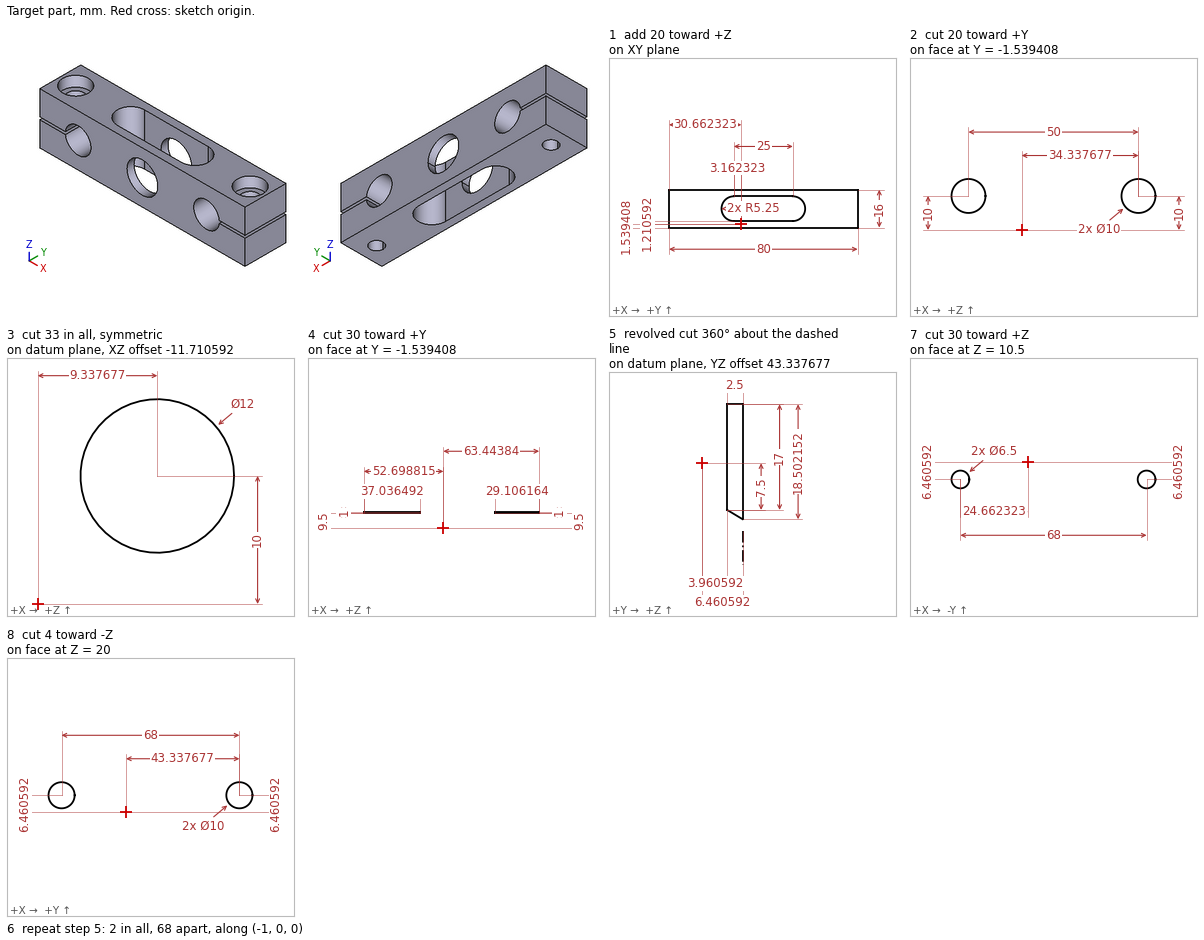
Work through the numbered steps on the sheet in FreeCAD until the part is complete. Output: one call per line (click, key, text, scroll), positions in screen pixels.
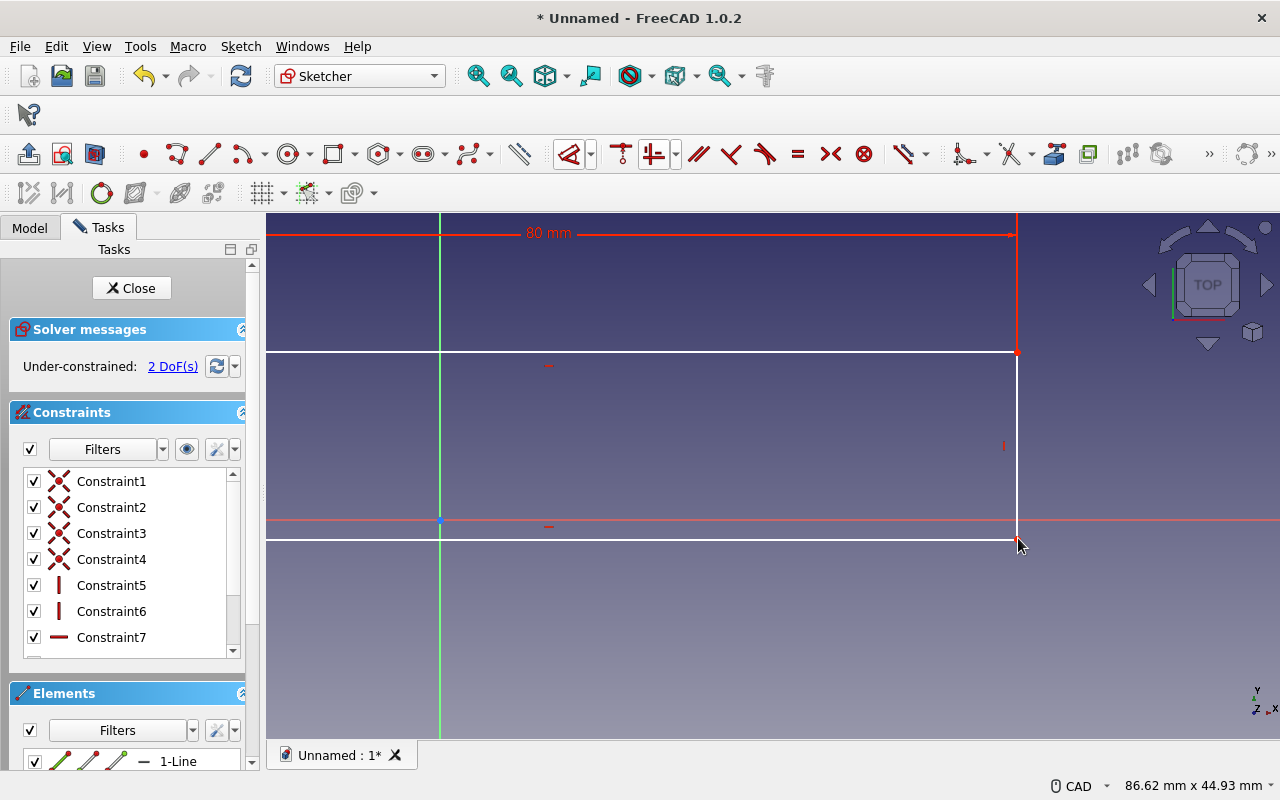
click(403, 444)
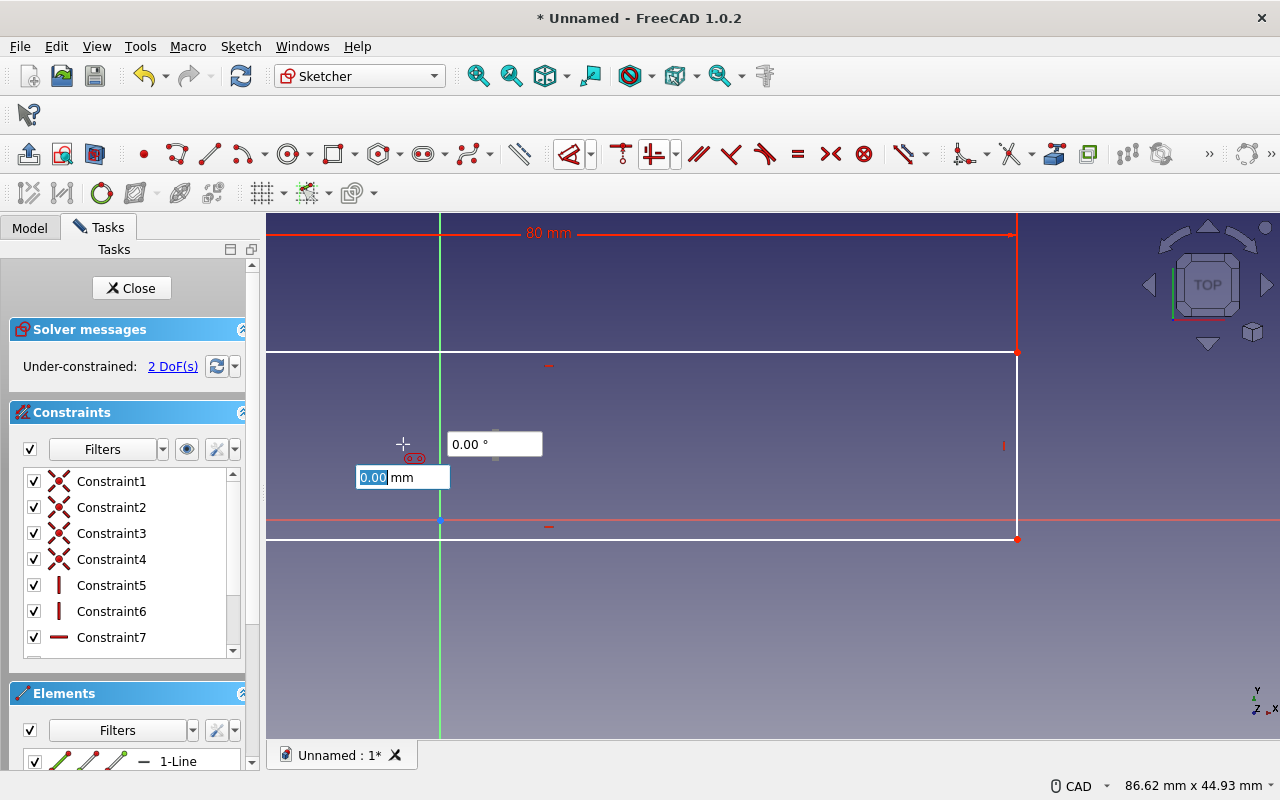
click(696, 444)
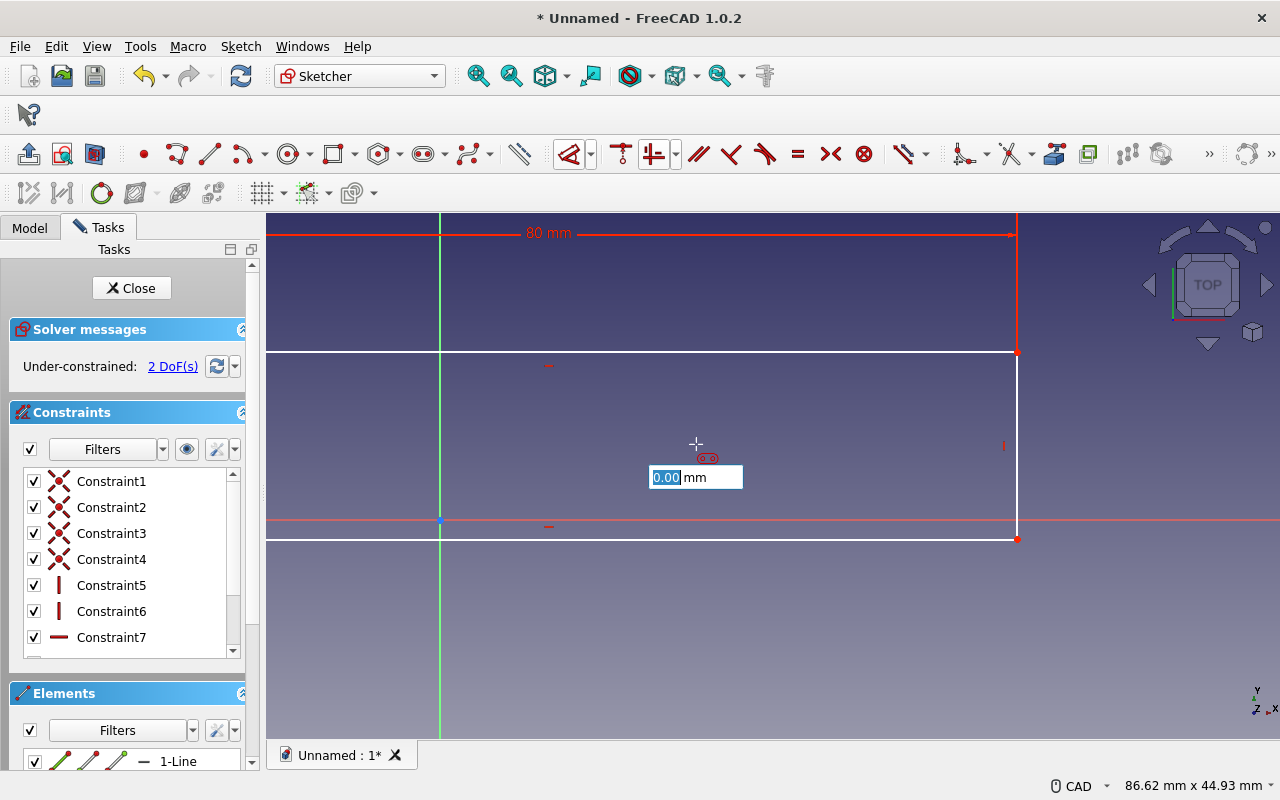
click(550, 383)
key(Escape)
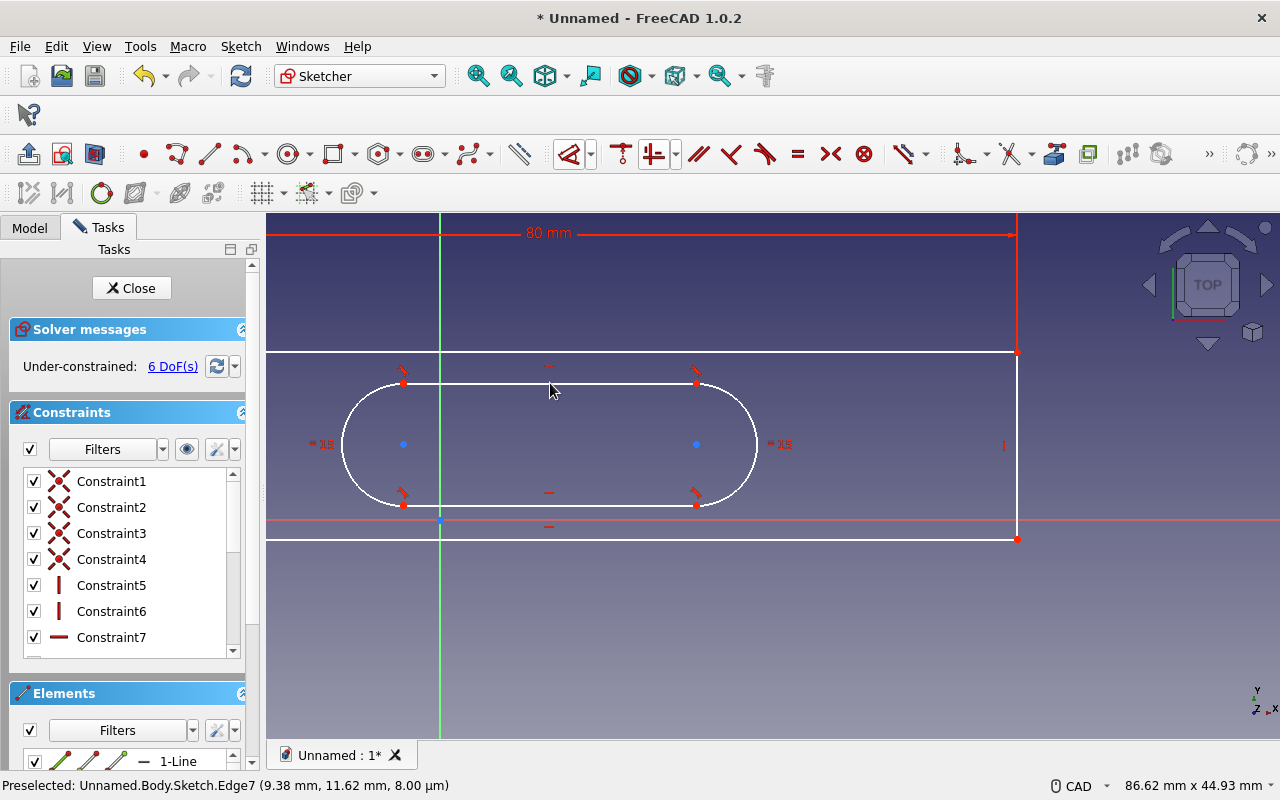
click(354, 409)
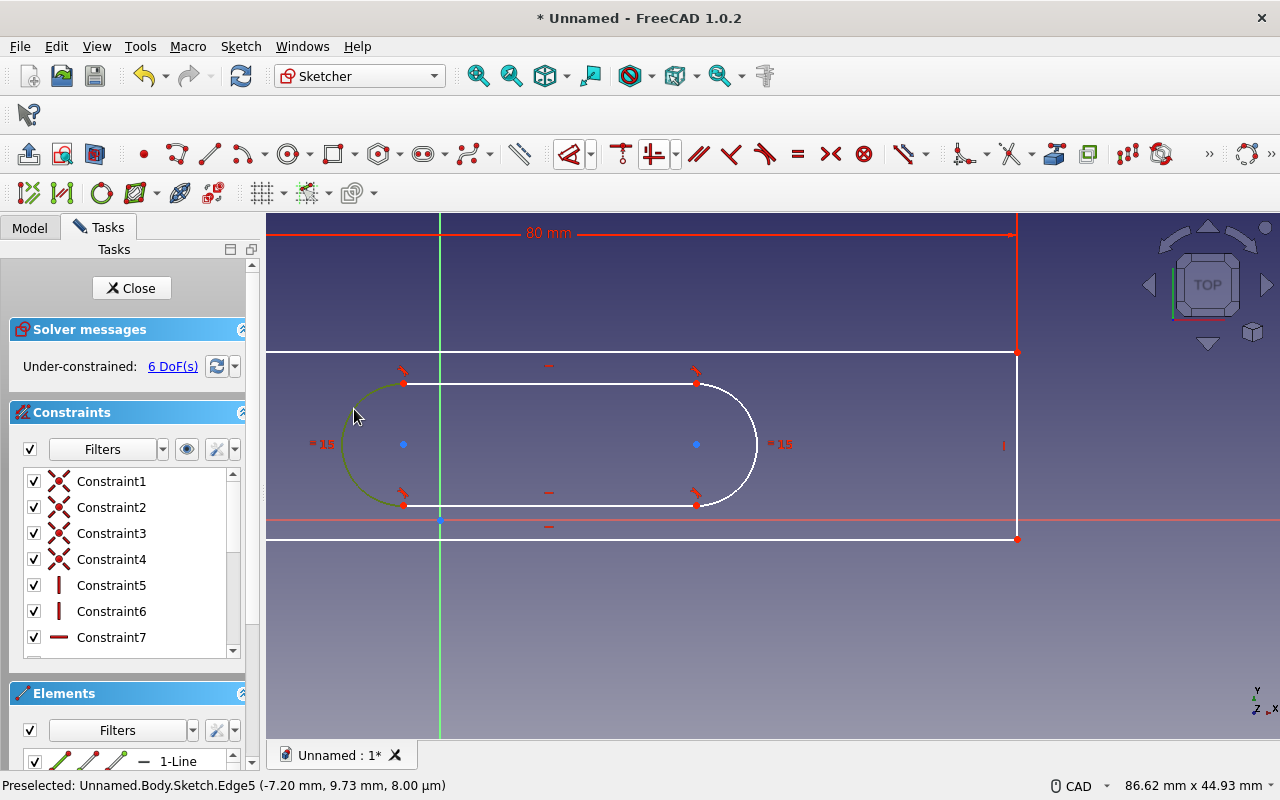
click(590, 154)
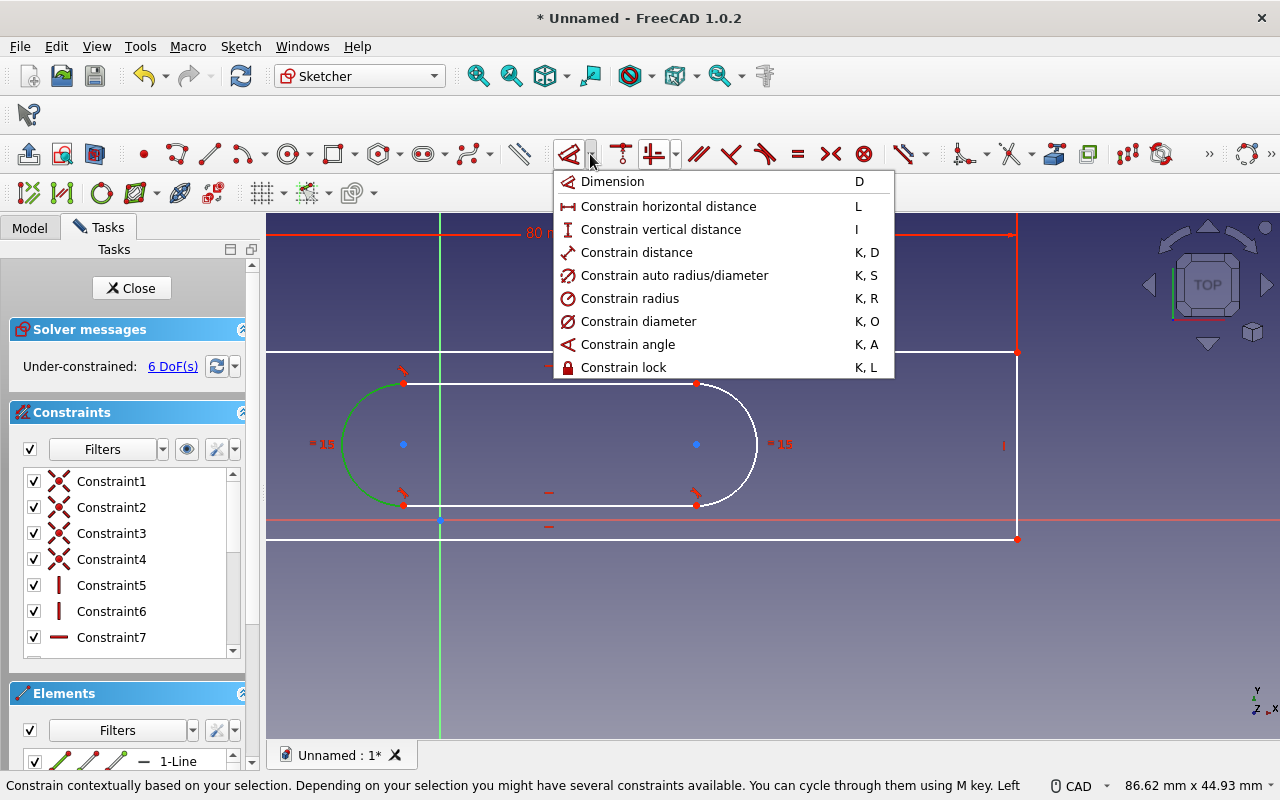
click(724, 298)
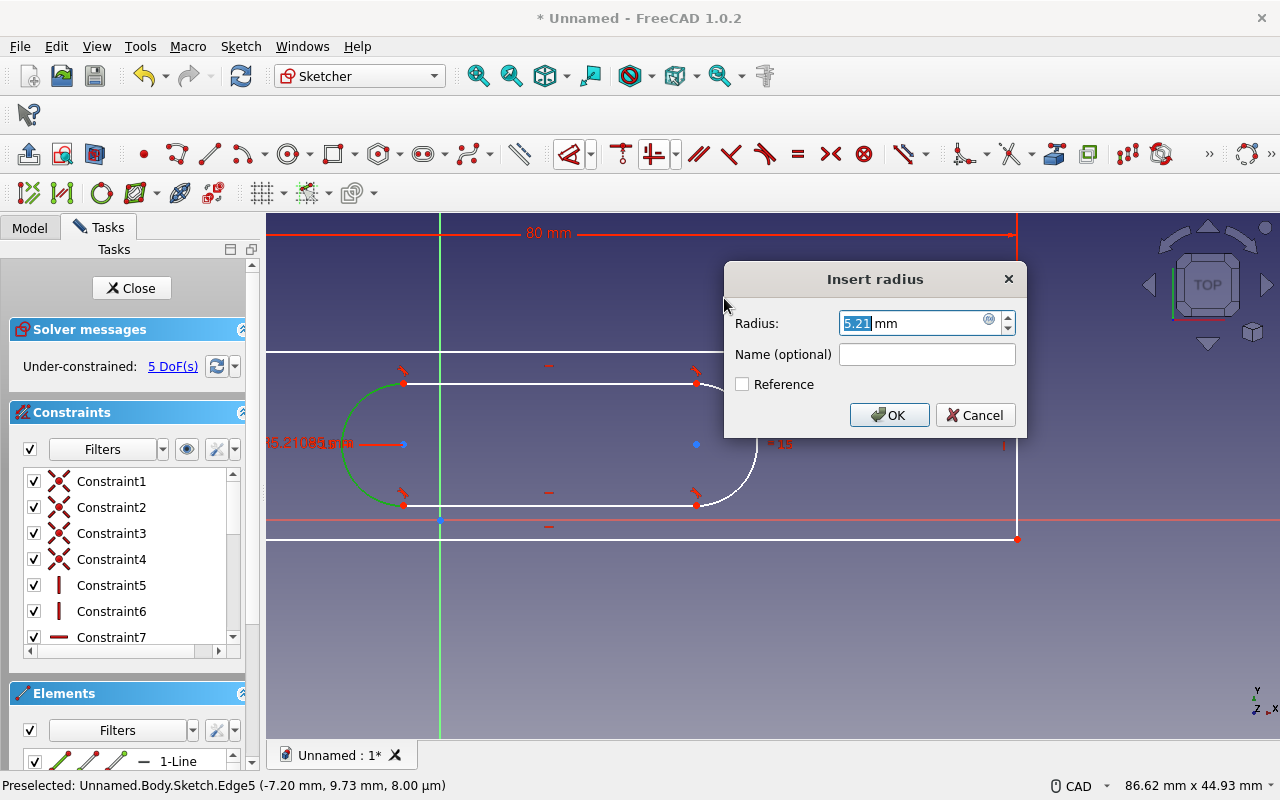
text(5.25)
key(Return)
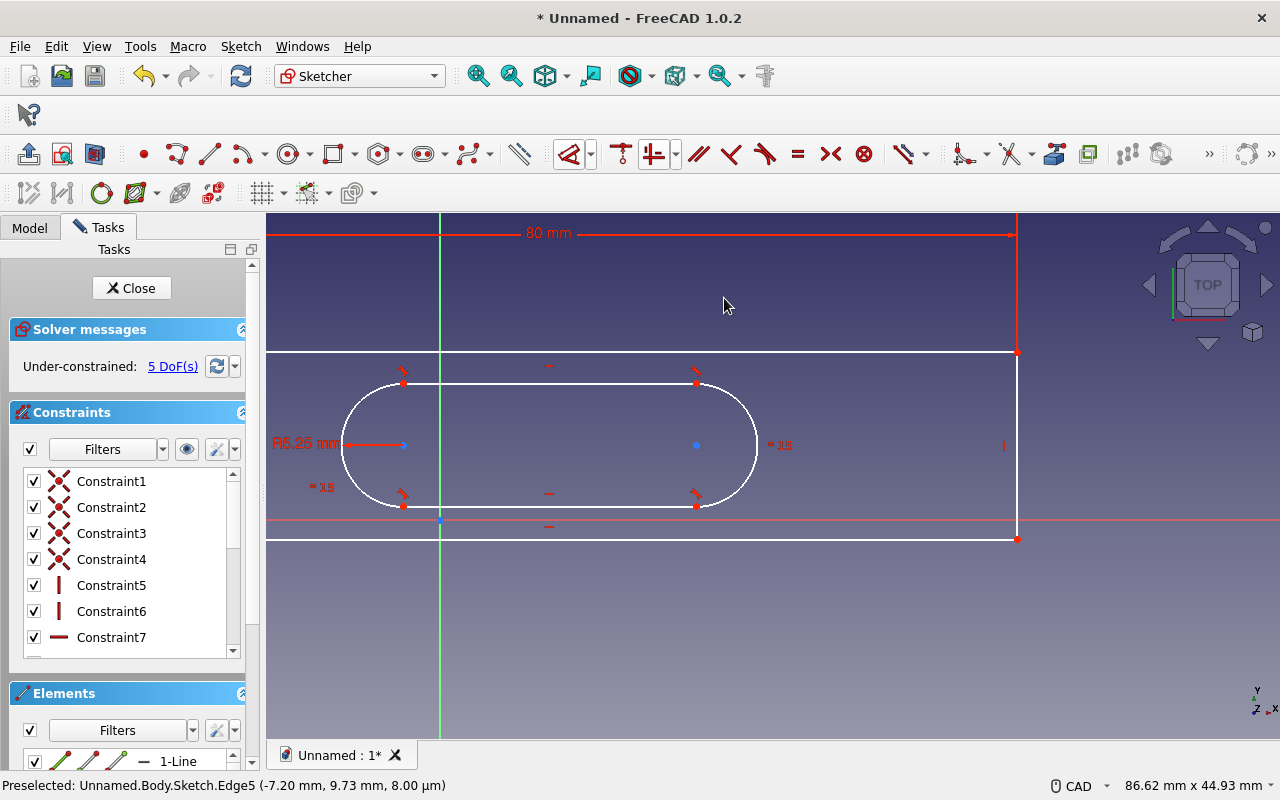
click(491, 384)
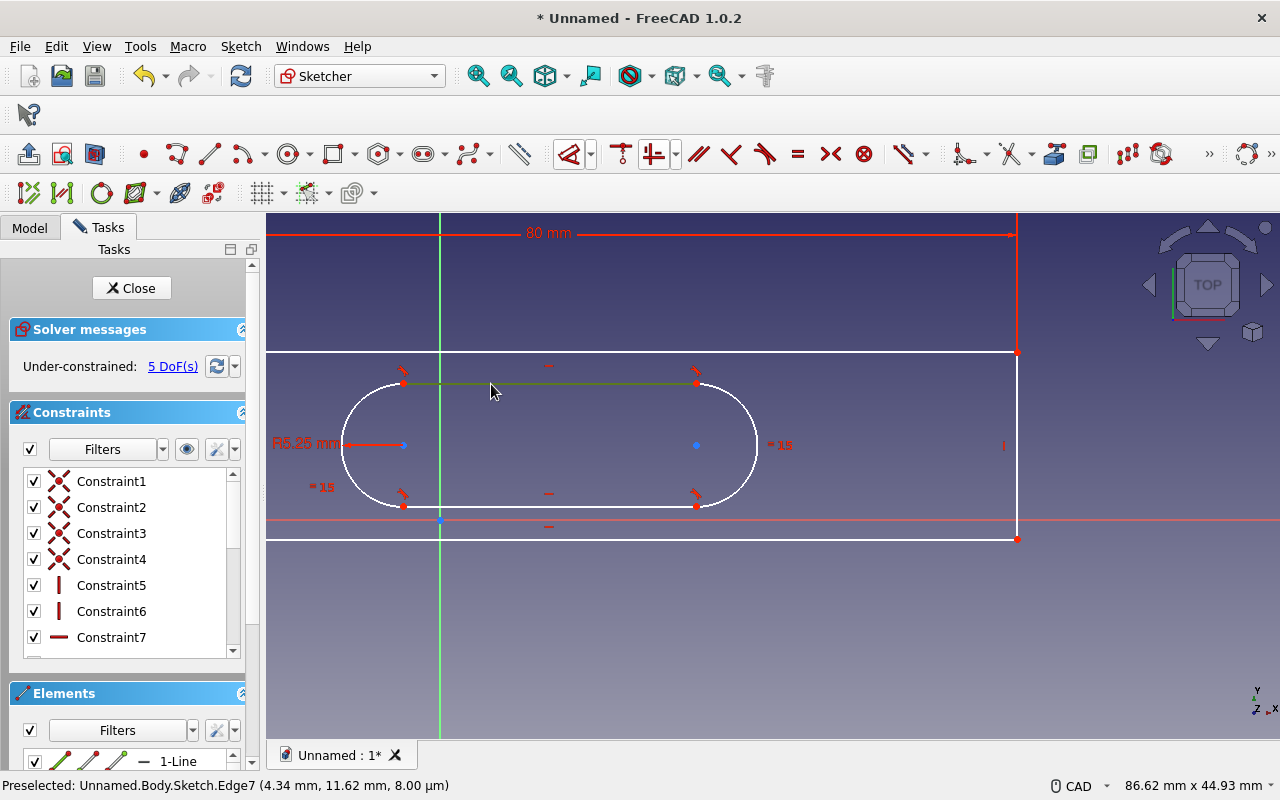
click(590, 154)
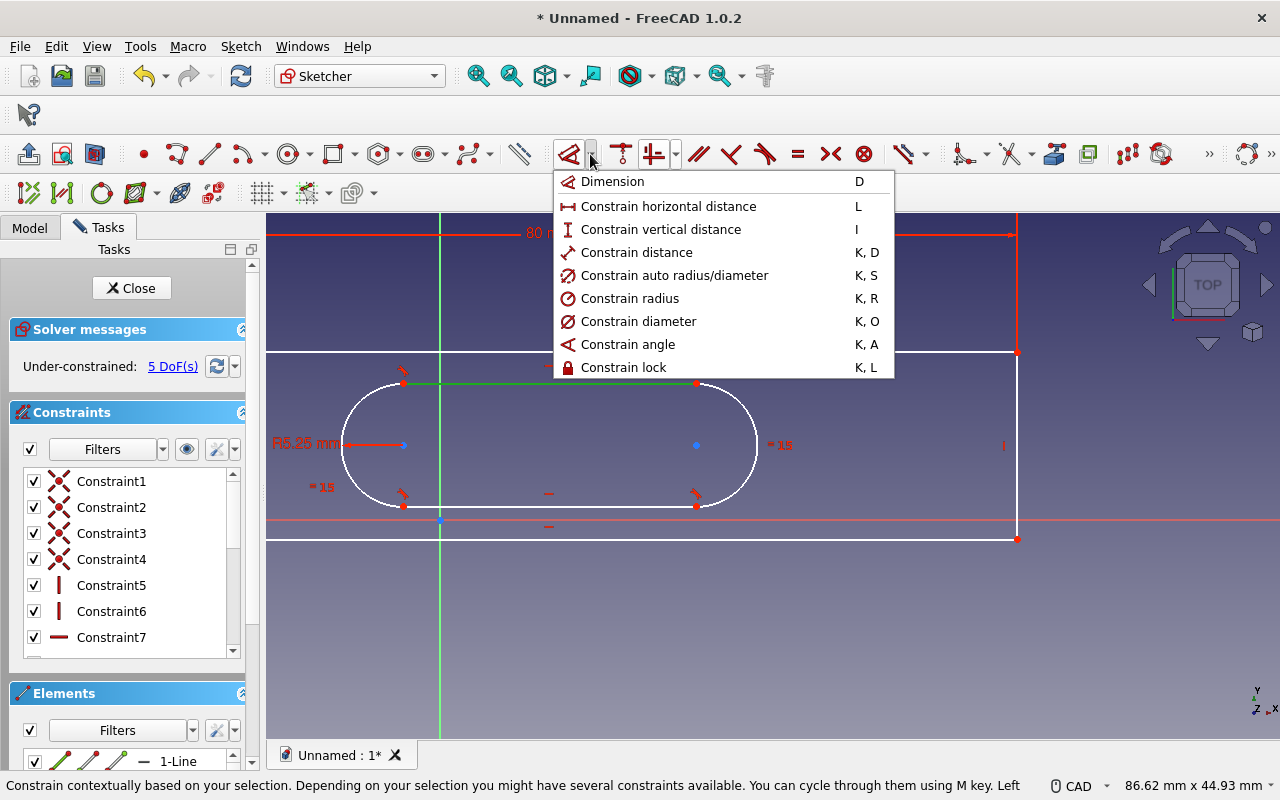
click(724, 206)